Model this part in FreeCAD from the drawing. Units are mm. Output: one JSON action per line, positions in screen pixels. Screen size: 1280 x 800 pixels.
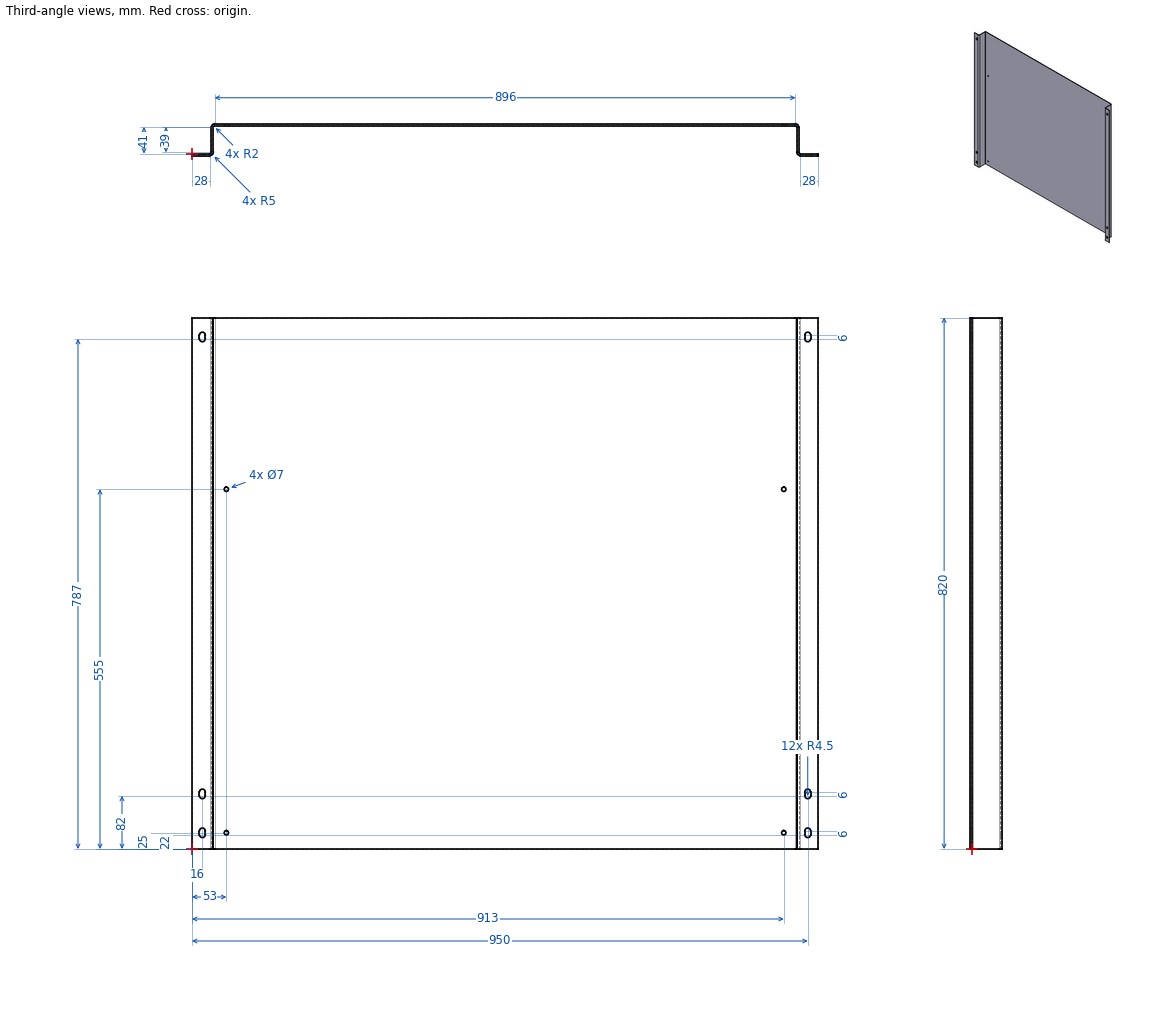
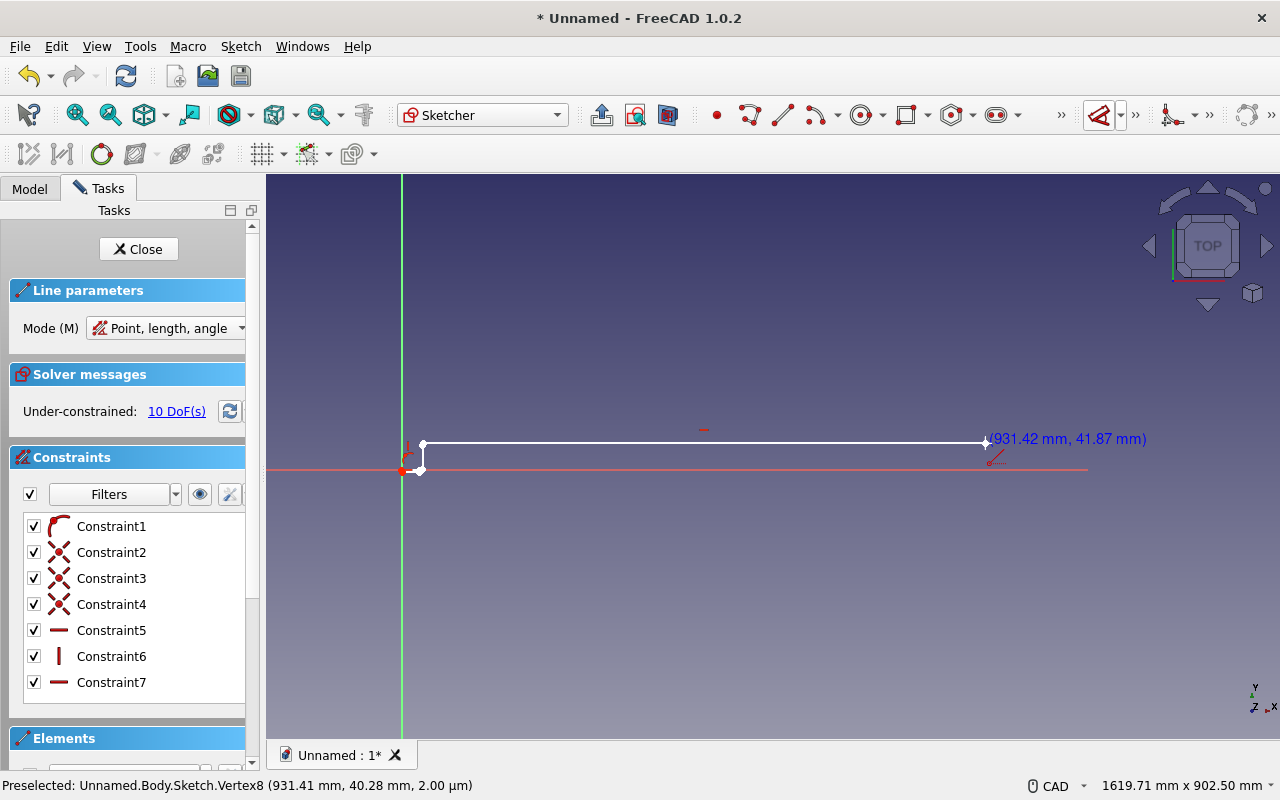
{"action": "scroll", "coordinate": [986, 445], "scroll_direction": "up", "scroll_amount": 11}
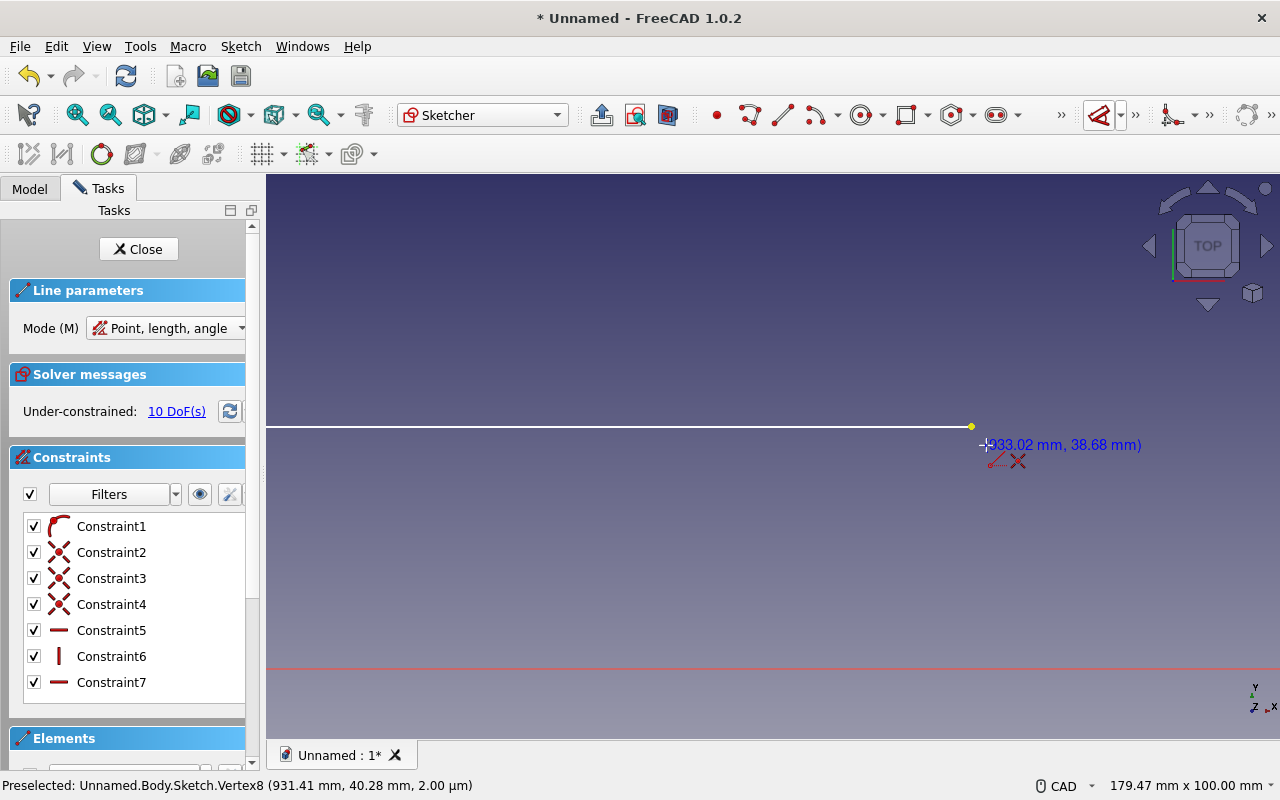
{"action": "left_click", "coordinate": [980, 437]}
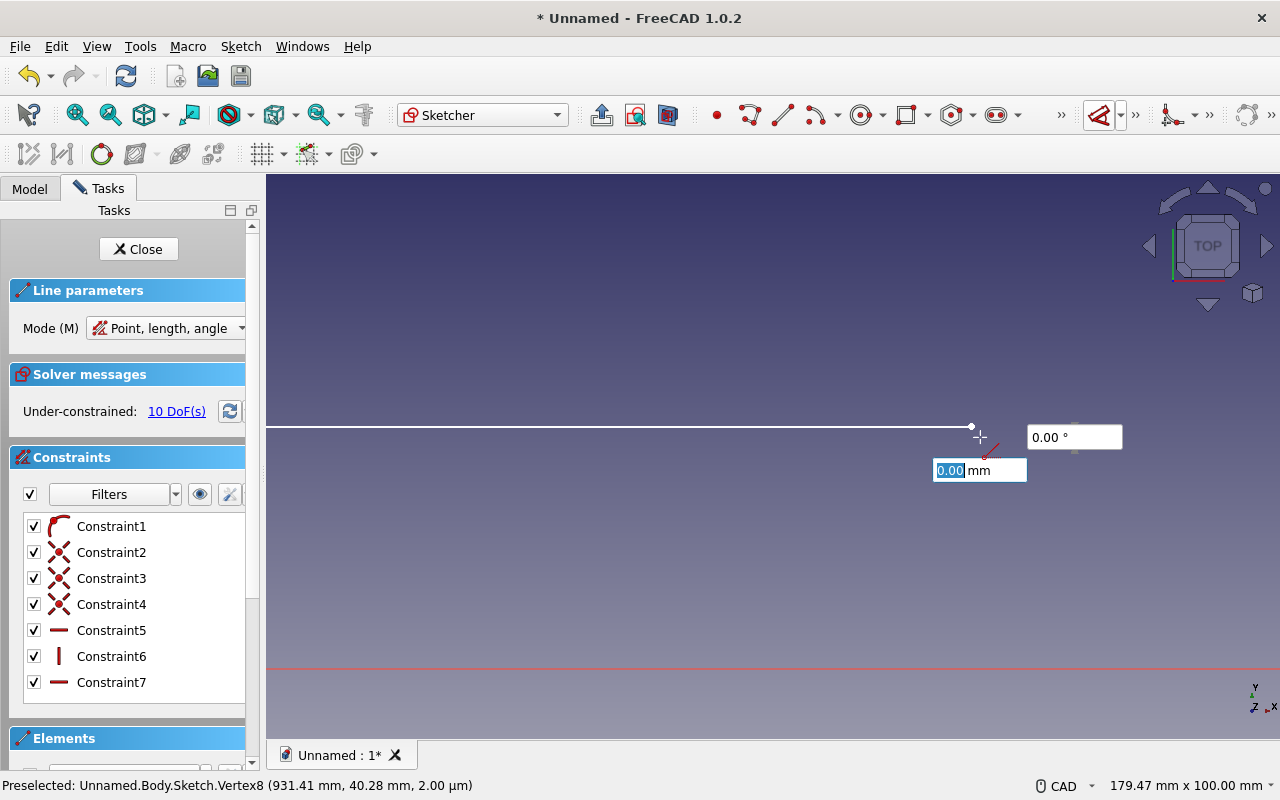
{"action": "scroll", "coordinate": [980, 657], "scroll_direction": "up", "scroll_amount": 2}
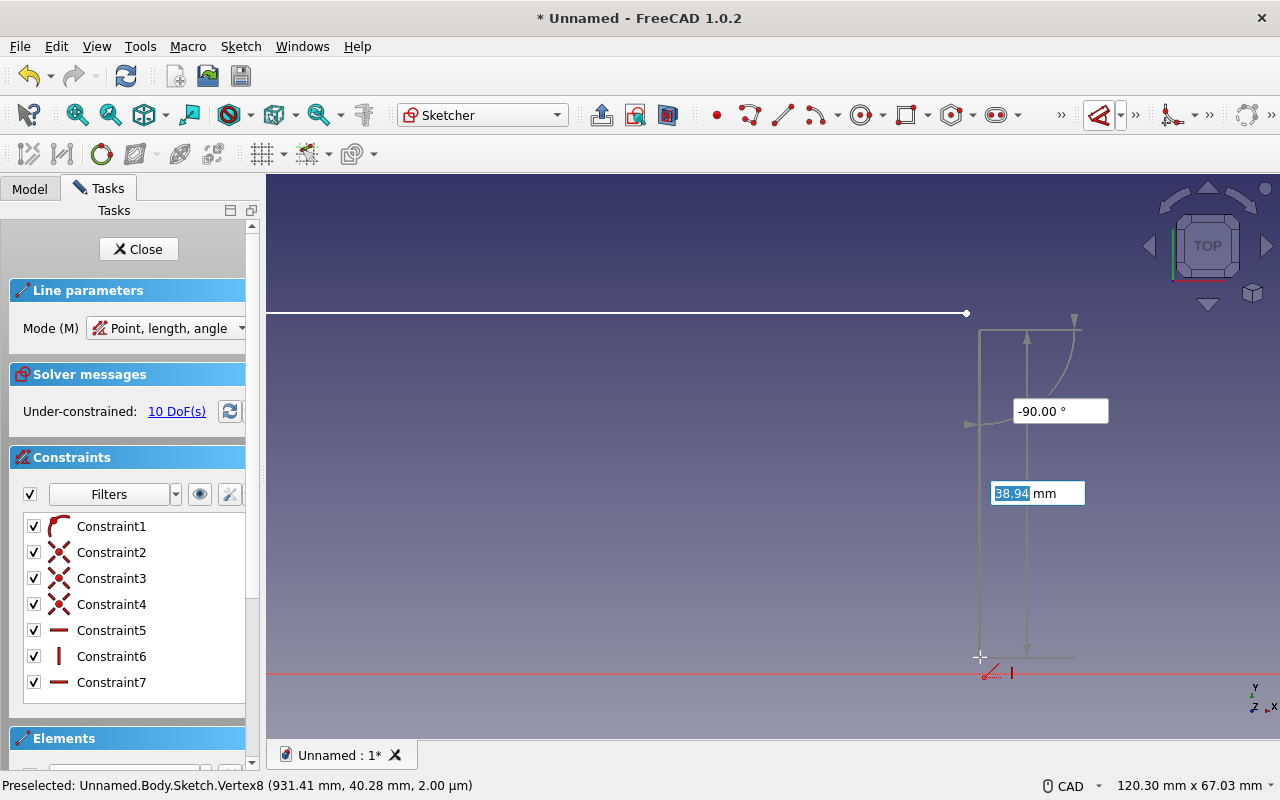
{"action": "left_click", "coordinate": [980, 657]}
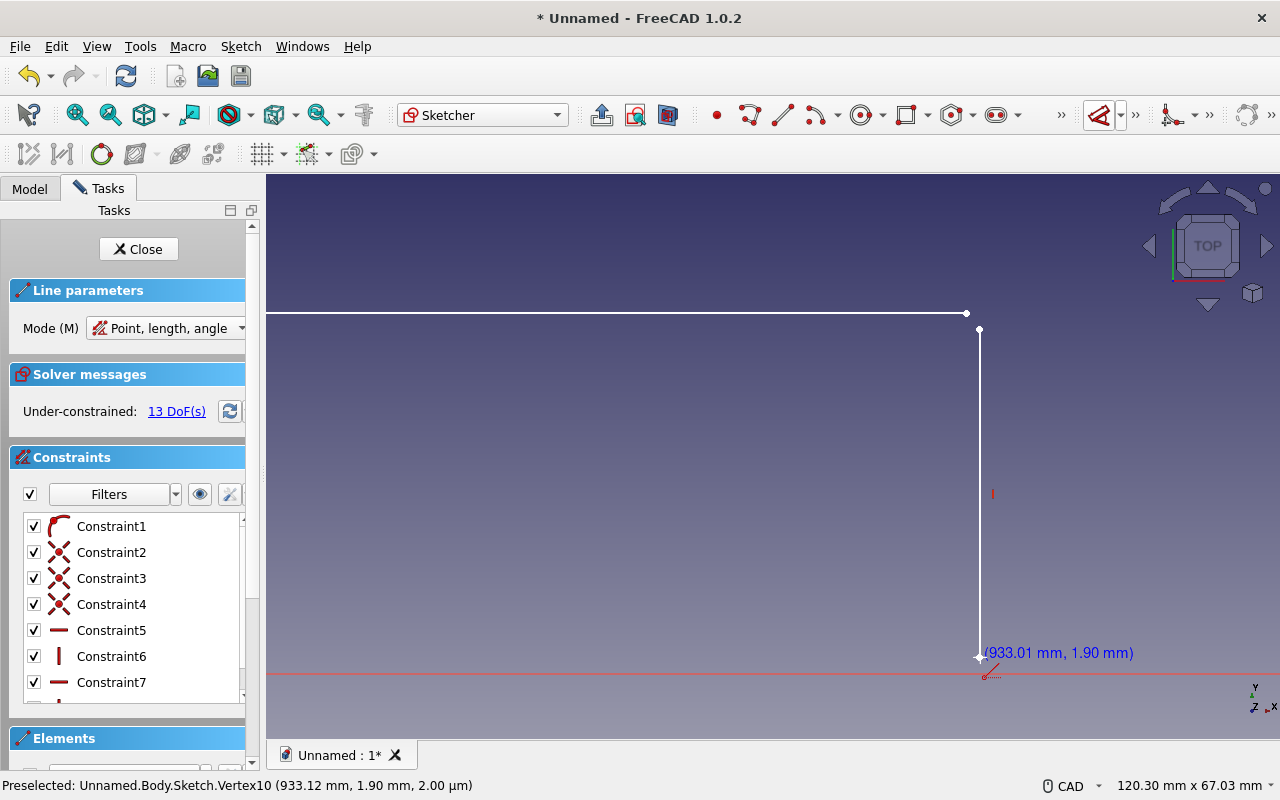
{"action": "left_click", "coordinate": [750, 116]}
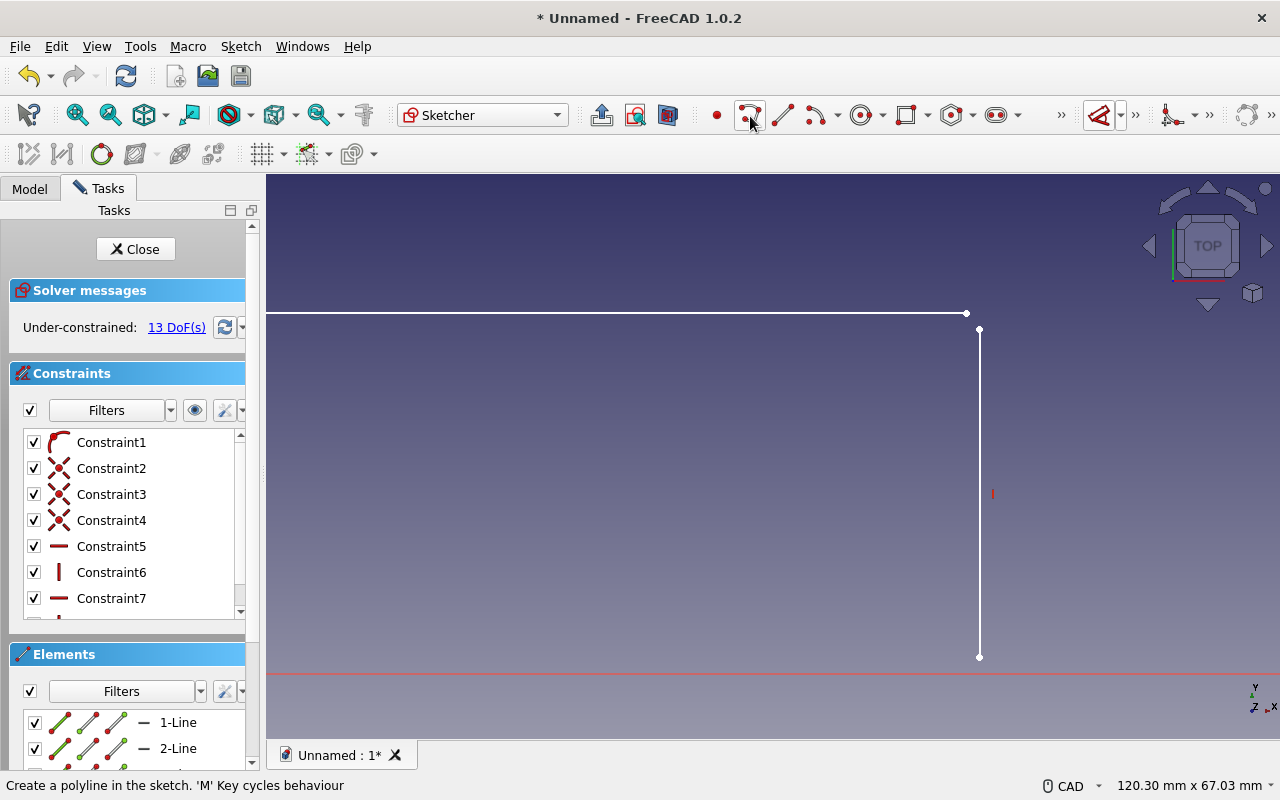
{"action": "left_click", "coordinate": [1022, 699]}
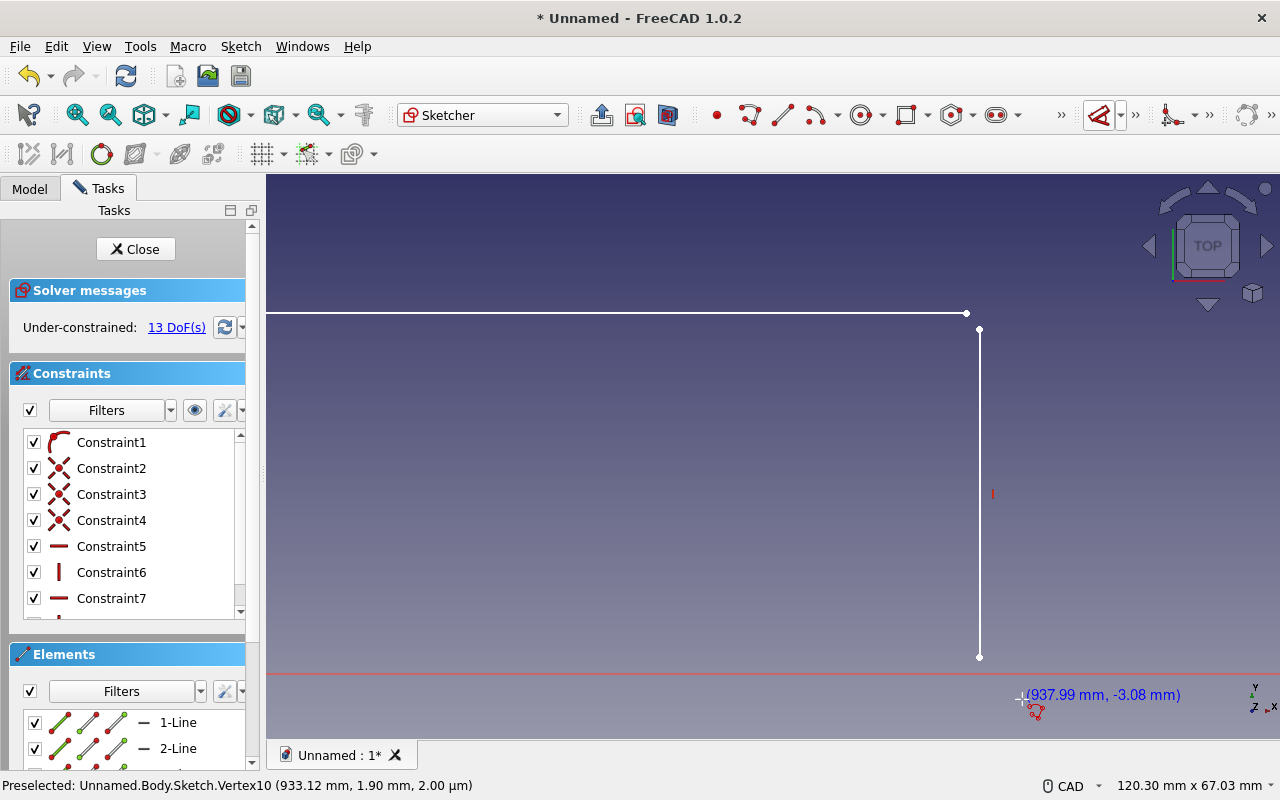
{"action": "scroll", "coordinate": [987, 454], "scroll_direction": "down", "scroll_amount": 13}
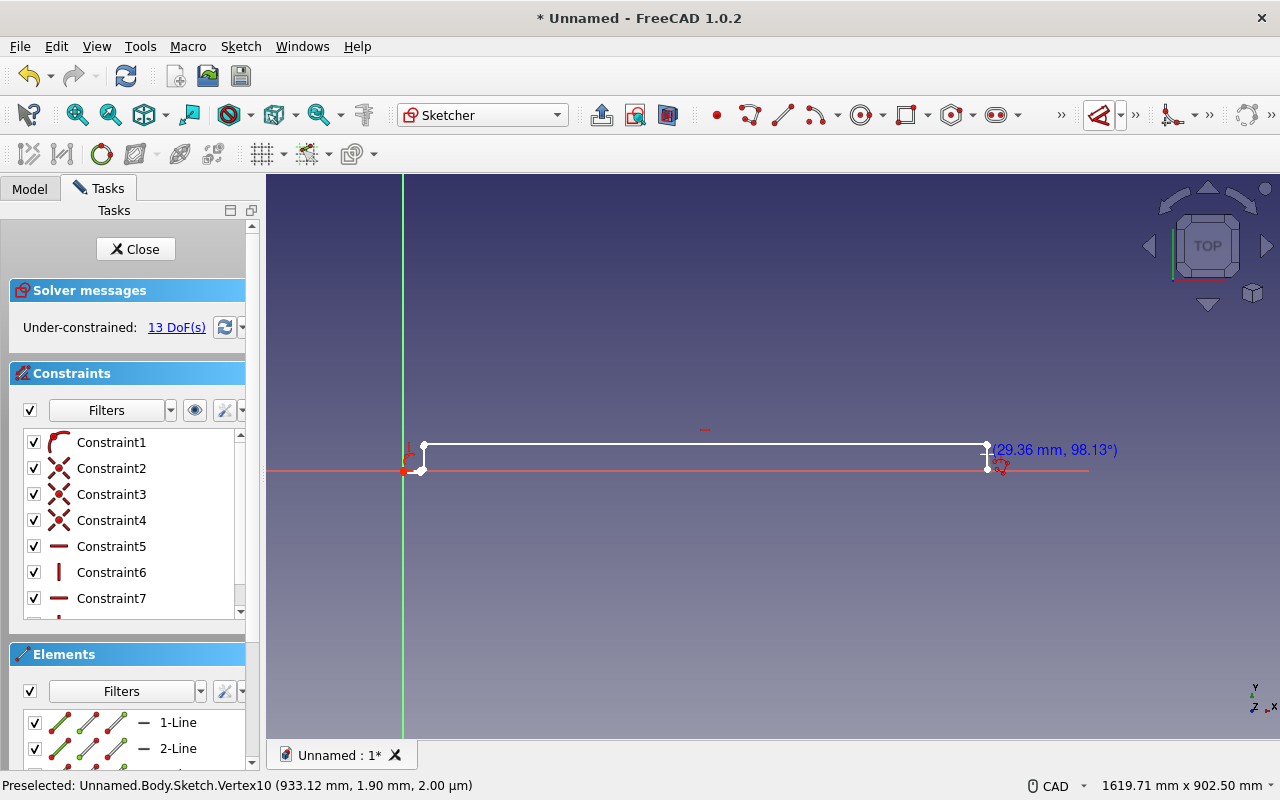
{"action": "scroll", "coordinate": [1008, 473], "scroll_direction": "up", "scroll_amount": 11}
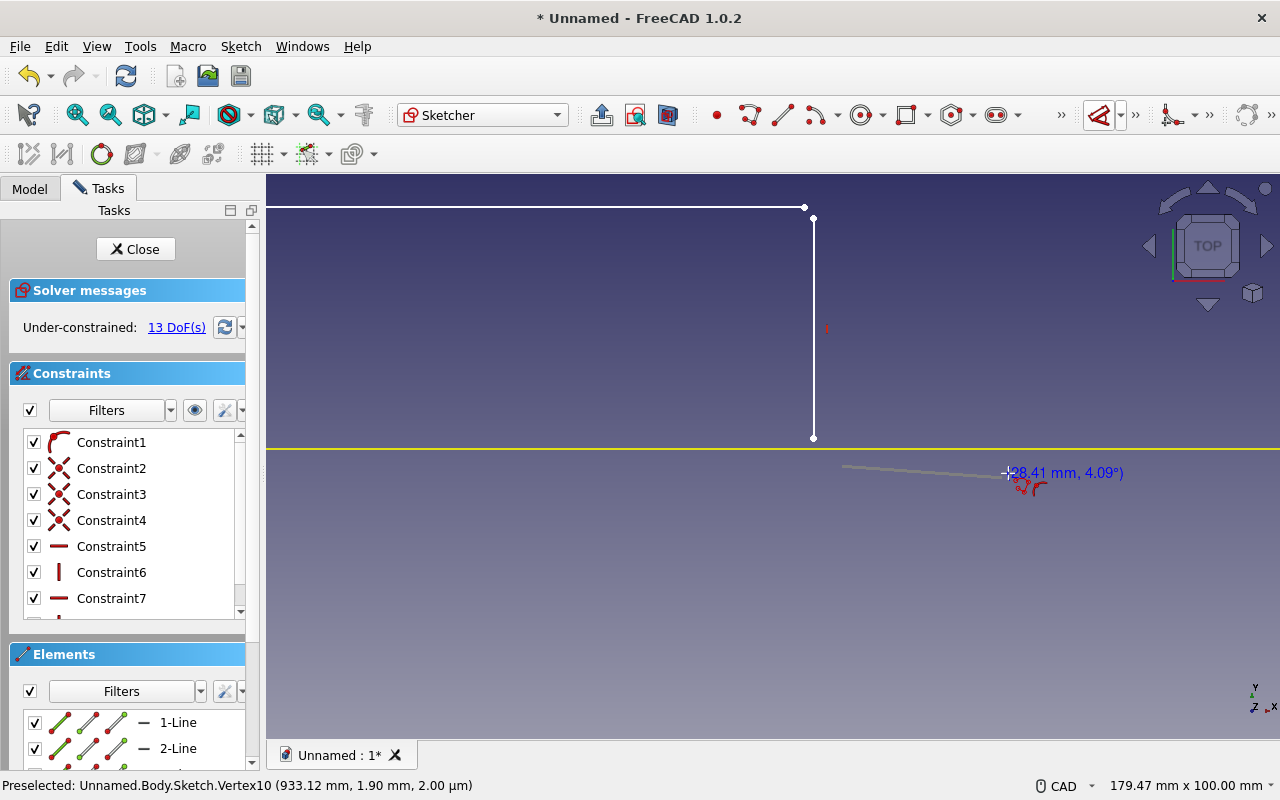
{"action": "left_click", "coordinate": [1000, 466]}
{"action": "left_click", "coordinate": [1000, 449]}
{"action": "left_click", "coordinate": [842, 440]}
{"action": "right_click", "coordinate": [842, 440]}